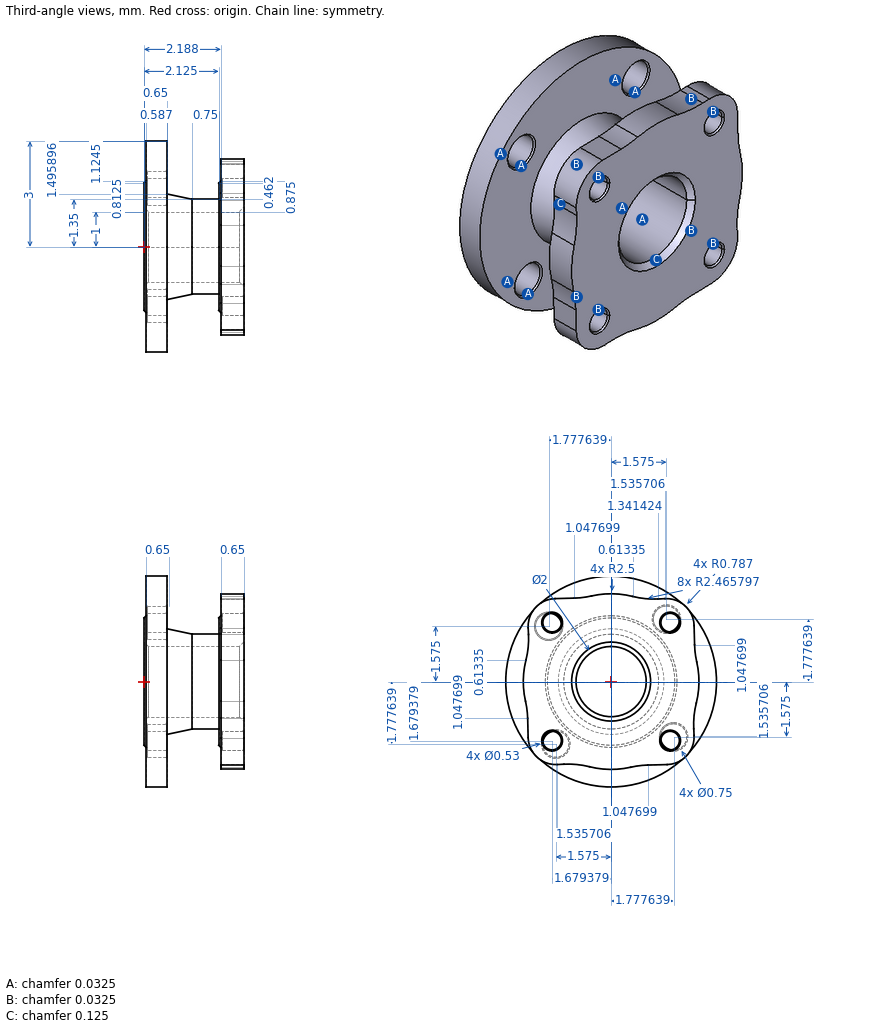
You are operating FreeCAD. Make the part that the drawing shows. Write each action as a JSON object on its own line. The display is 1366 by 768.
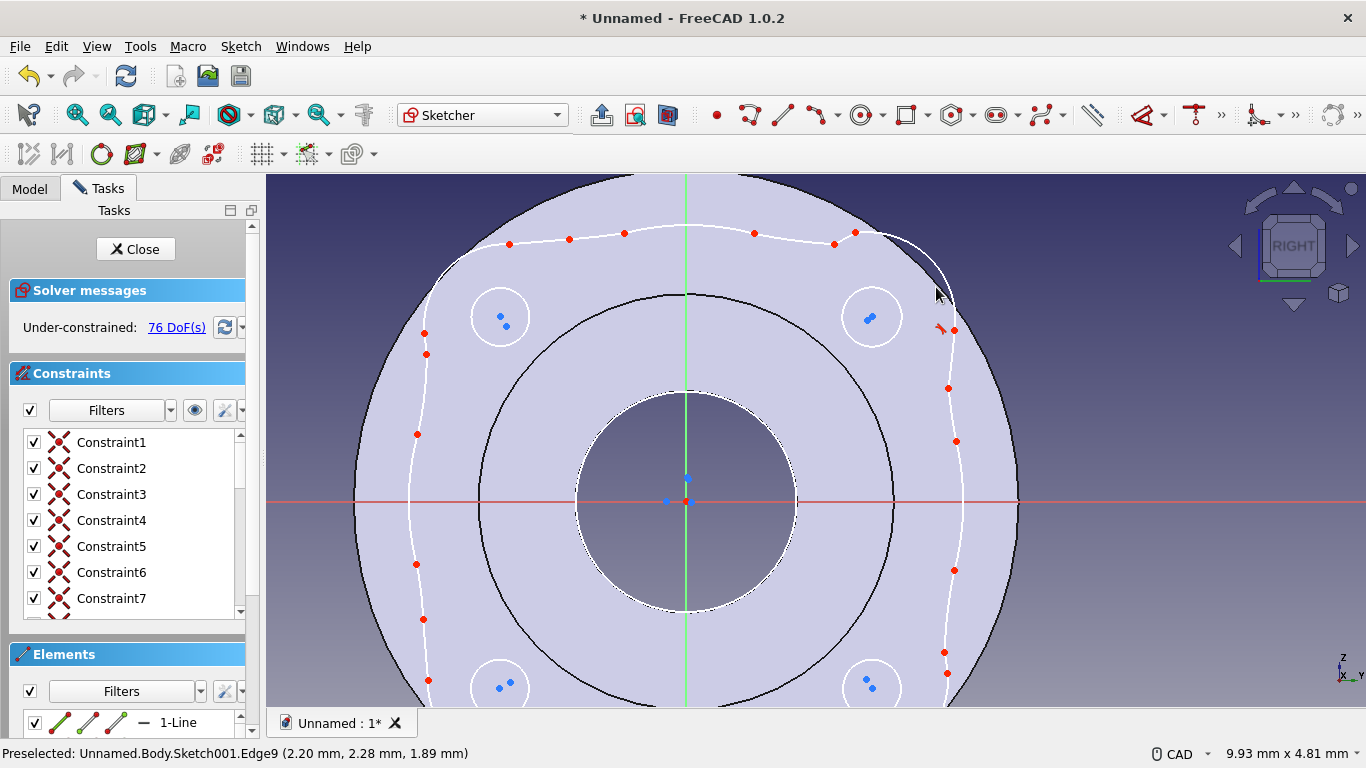
{"action": "left_click", "coordinate": [950, 371]}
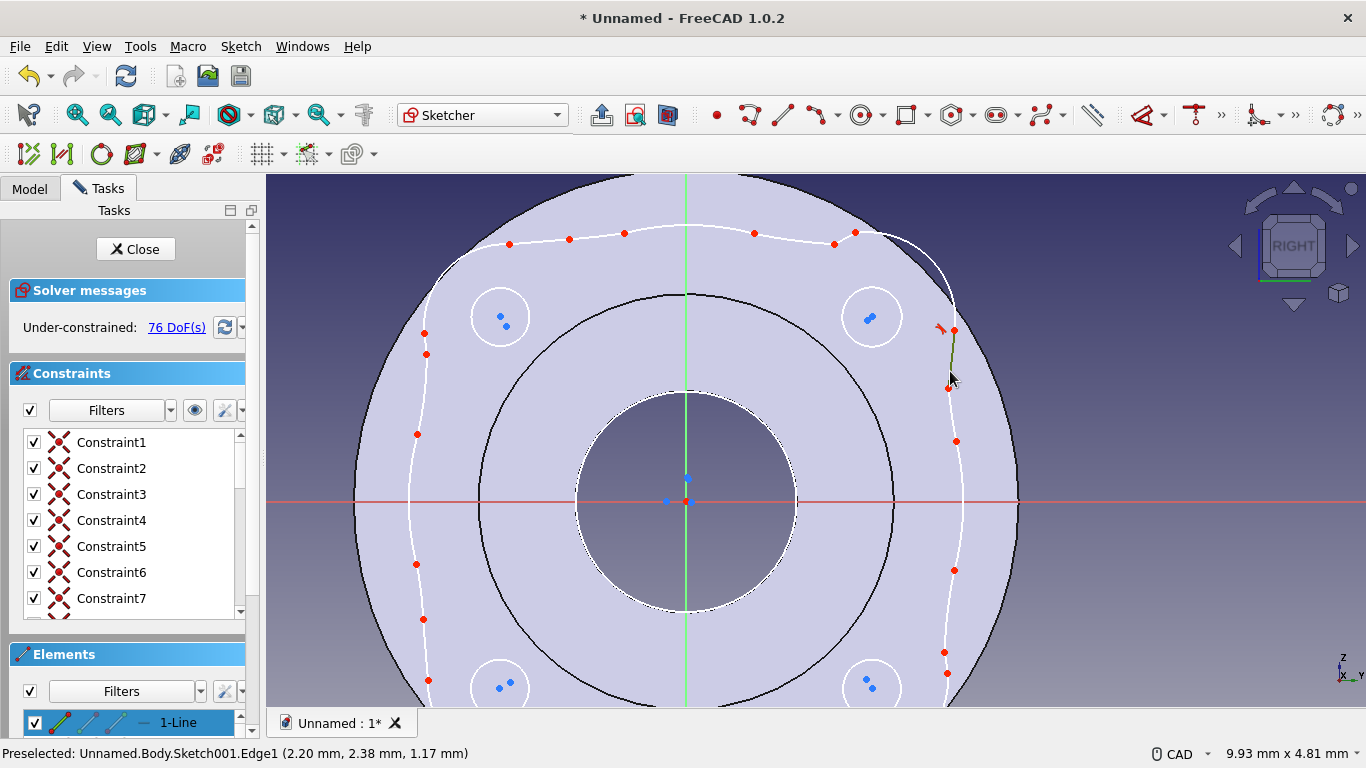
{"action": "left_click", "coordinate": [950, 404]}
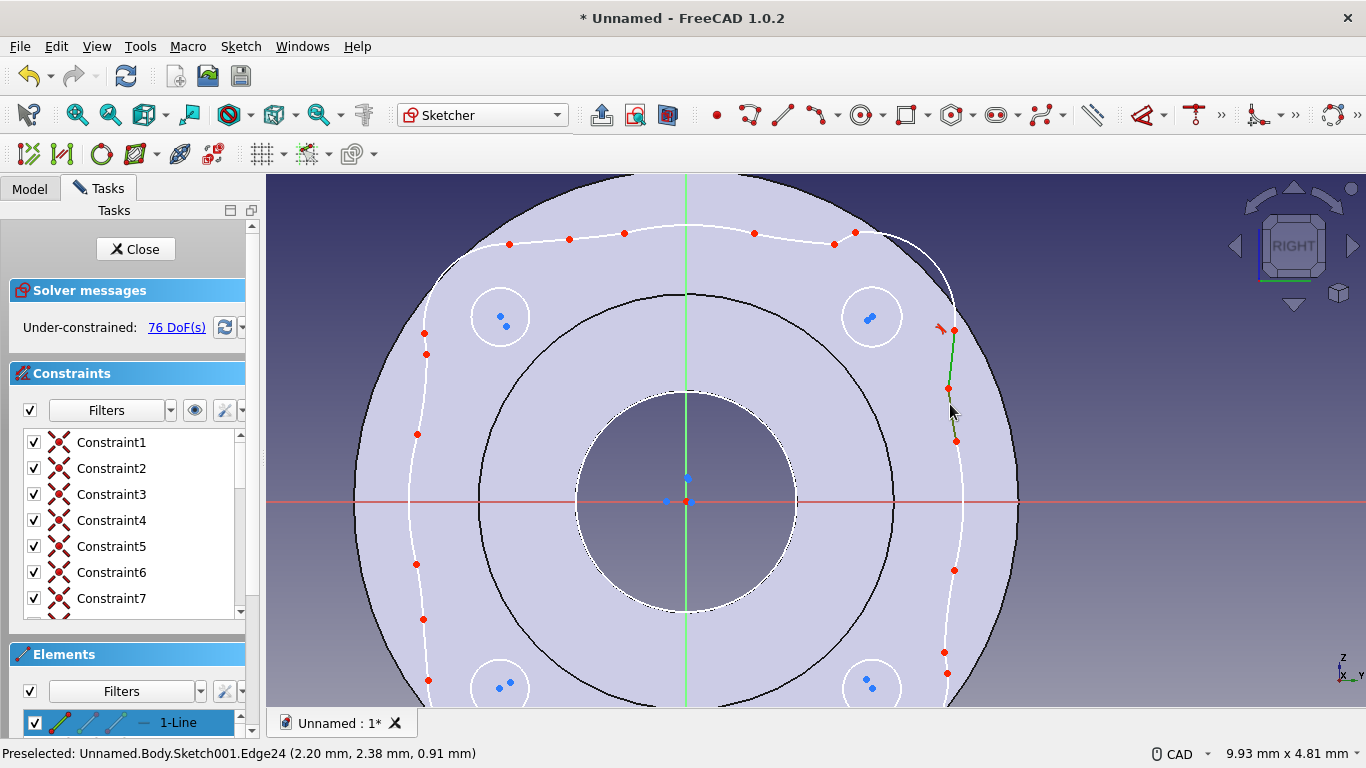
{"action": "key", "text": "t"}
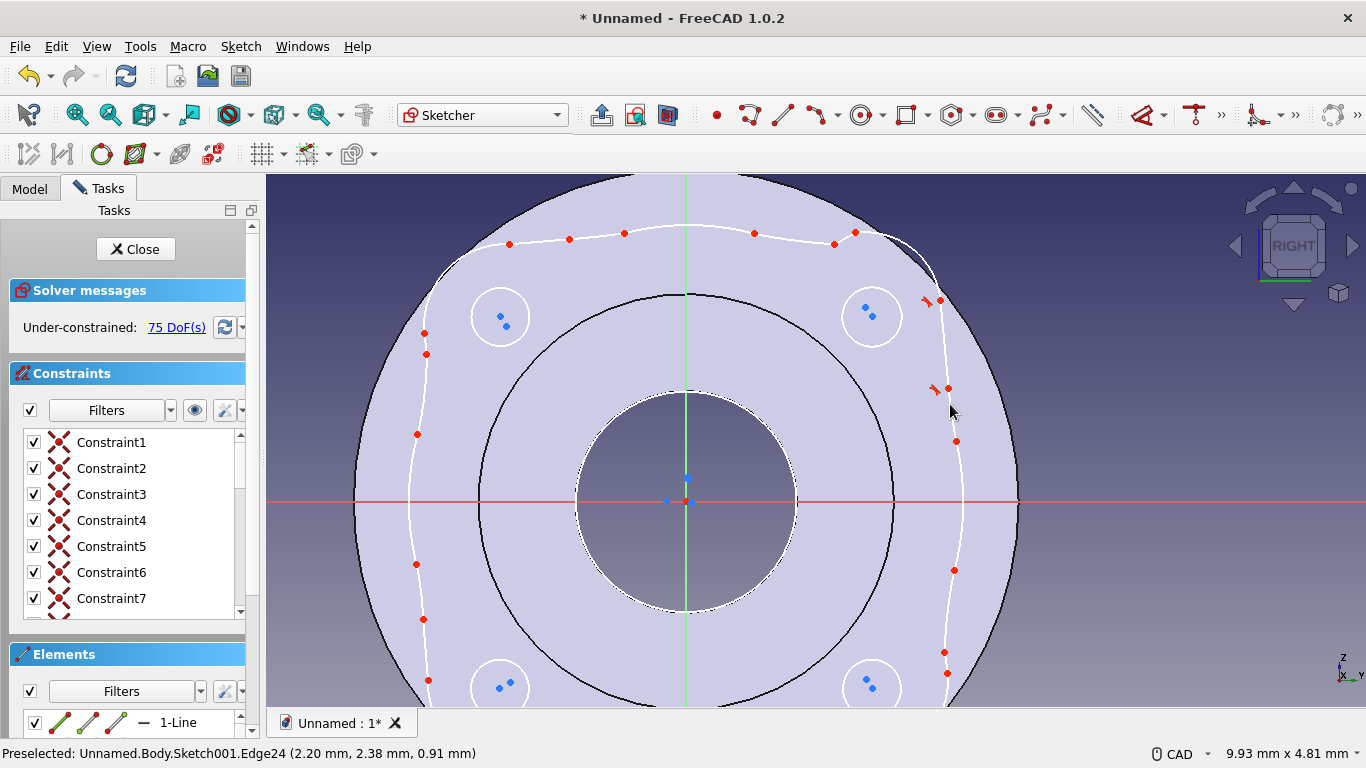
{"action": "scroll", "coordinate": [847, 237], "scroll_direction": "up", "scroll_amount": 2}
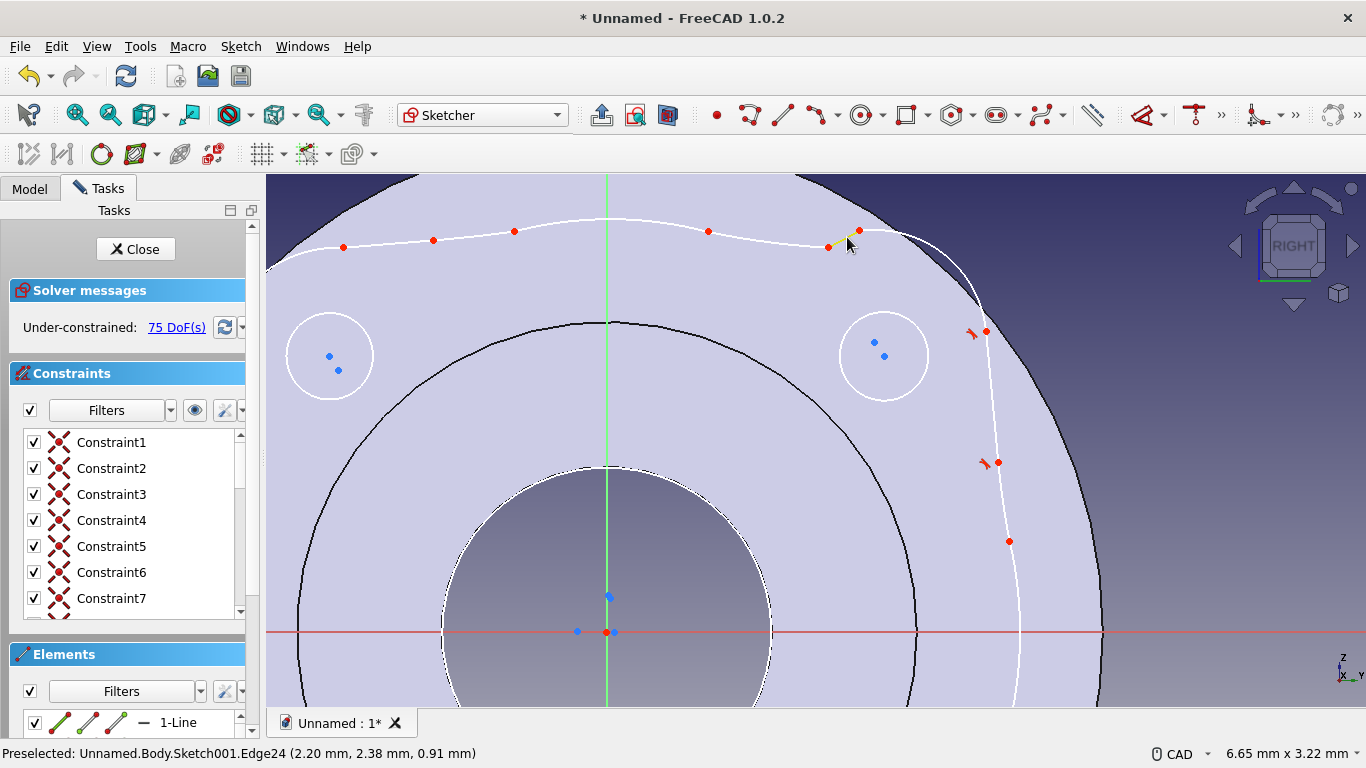
{"action": "left_click", "coordinate": [847, 238]}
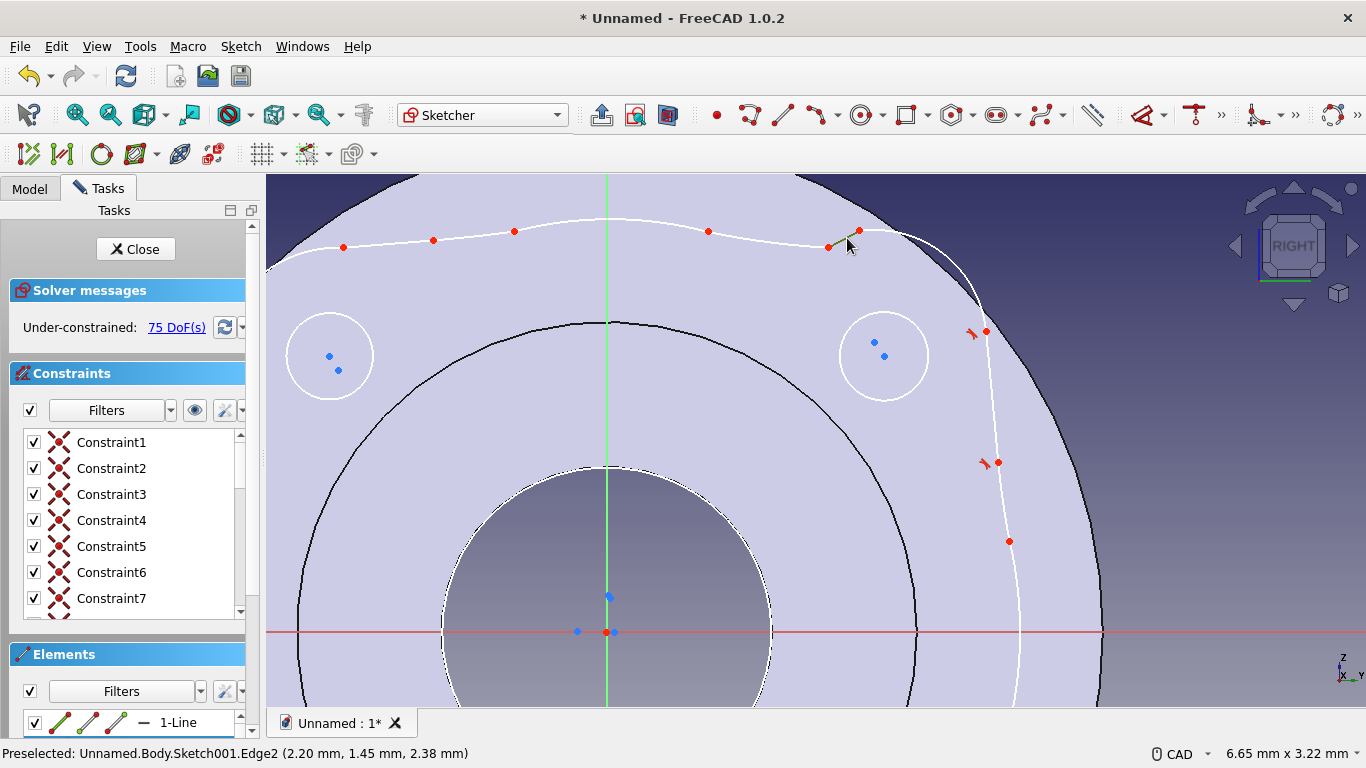
{"action": "left_click", "coordinate": [969, 281]}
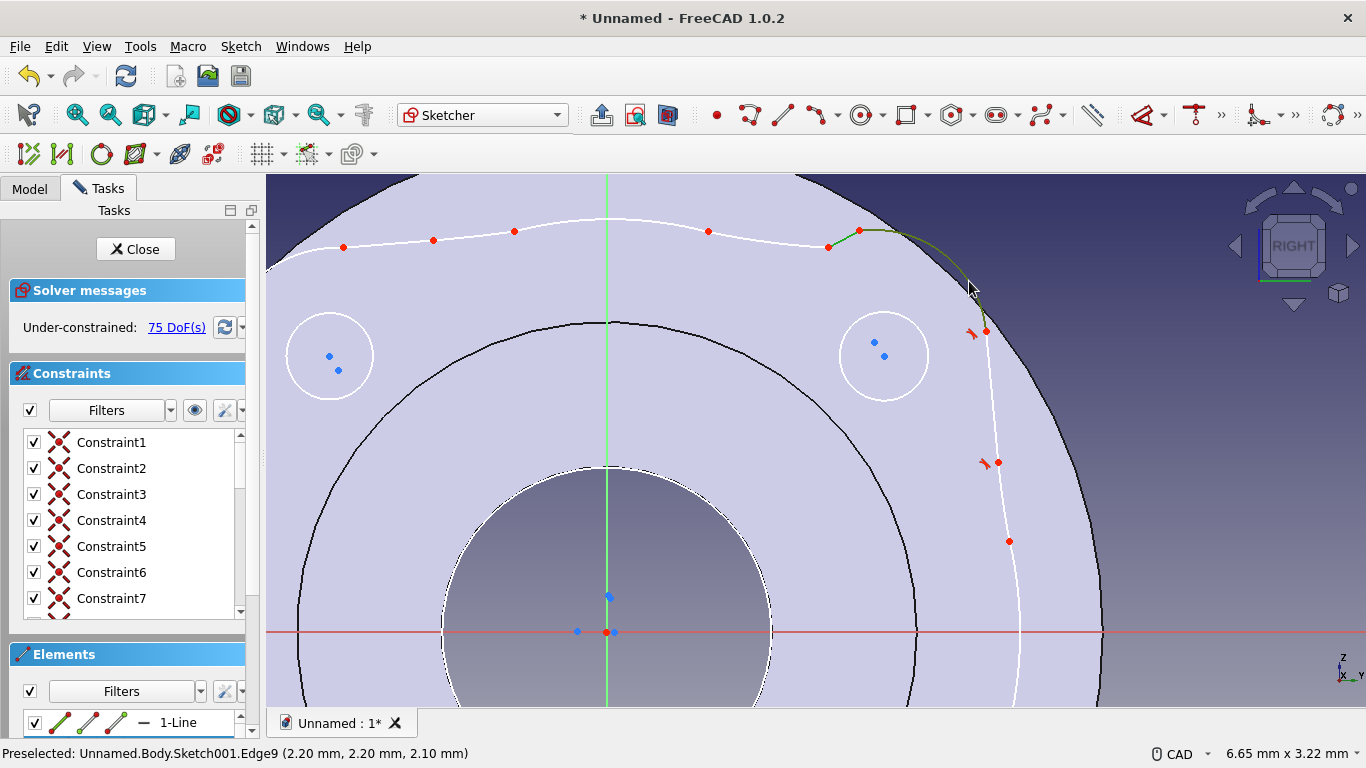
{"action": "key", "text": "t"}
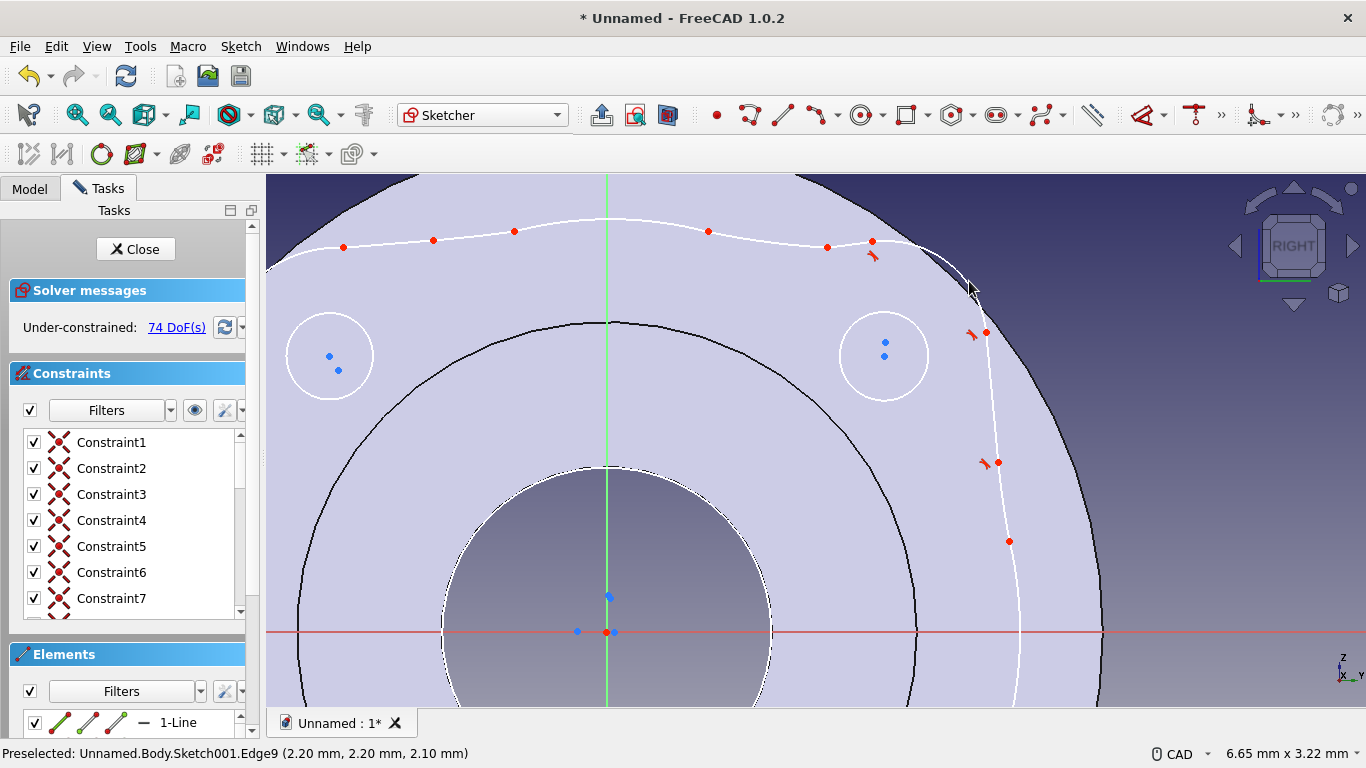
{"action": "left_click", "coordinate": [859, 244]}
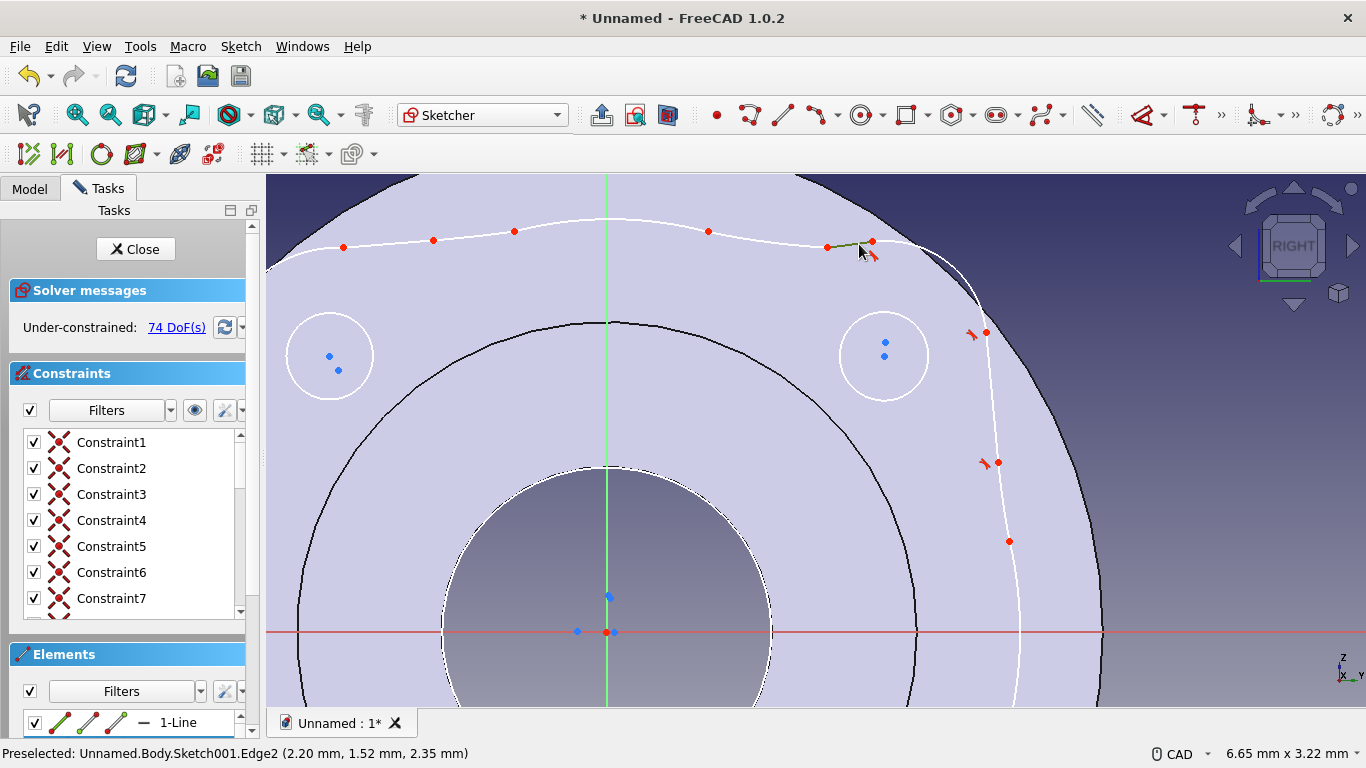
{"action": "left_click", "coordinate": [744, 239]}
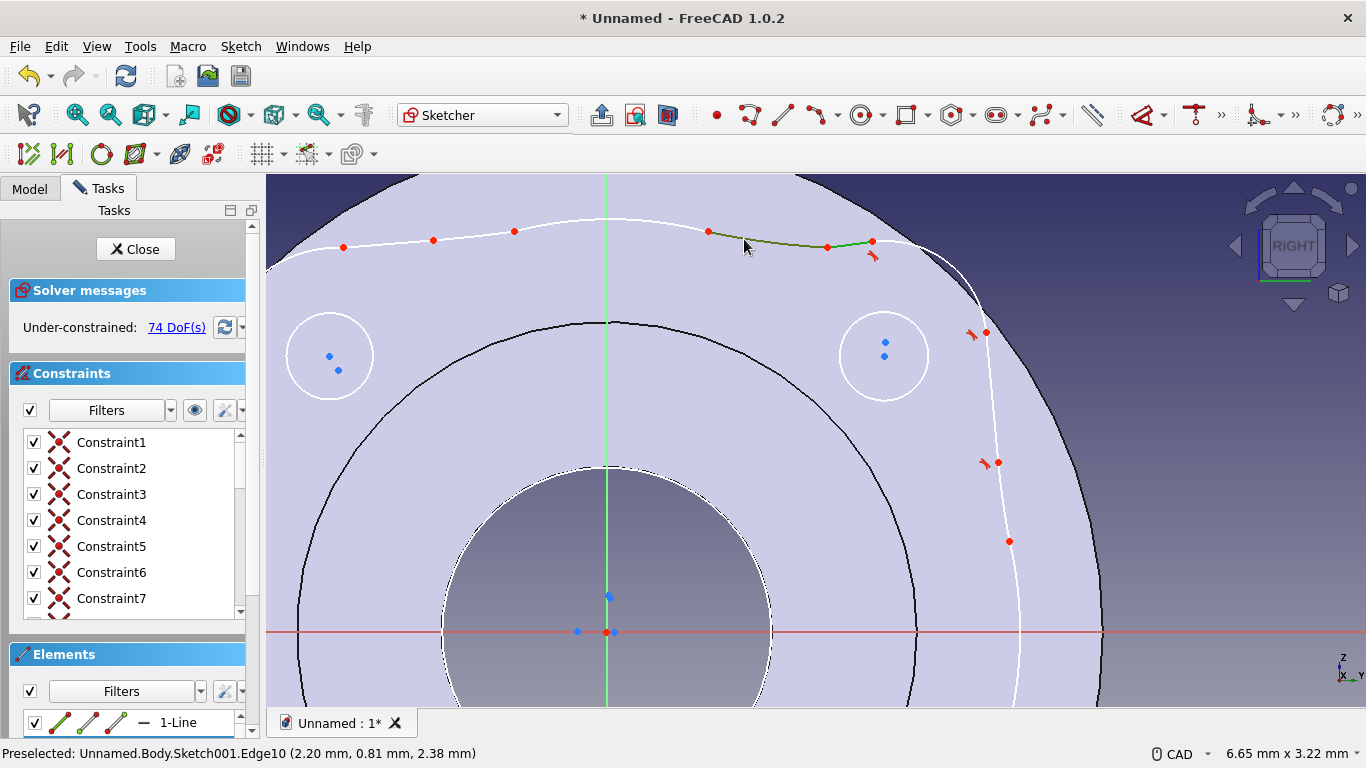
{"action": "key", "text": "t"}